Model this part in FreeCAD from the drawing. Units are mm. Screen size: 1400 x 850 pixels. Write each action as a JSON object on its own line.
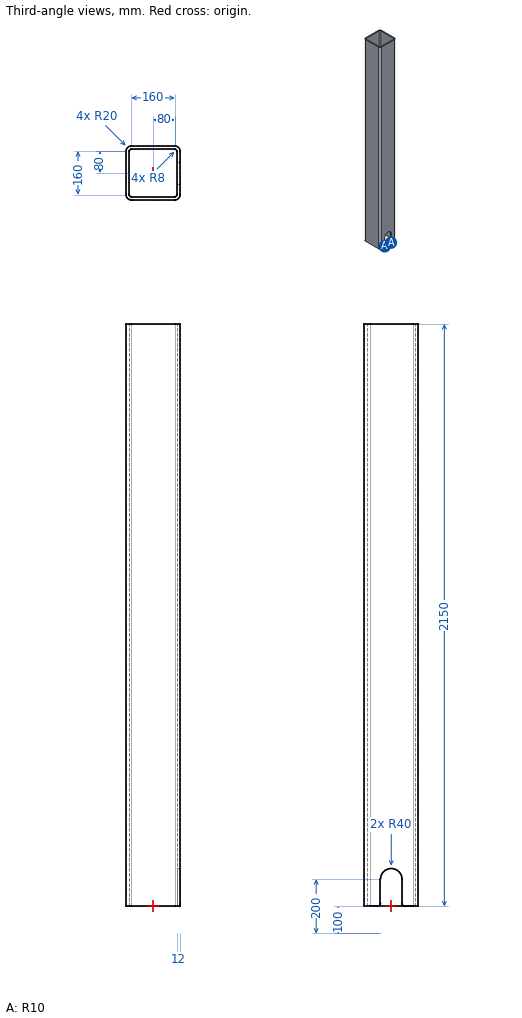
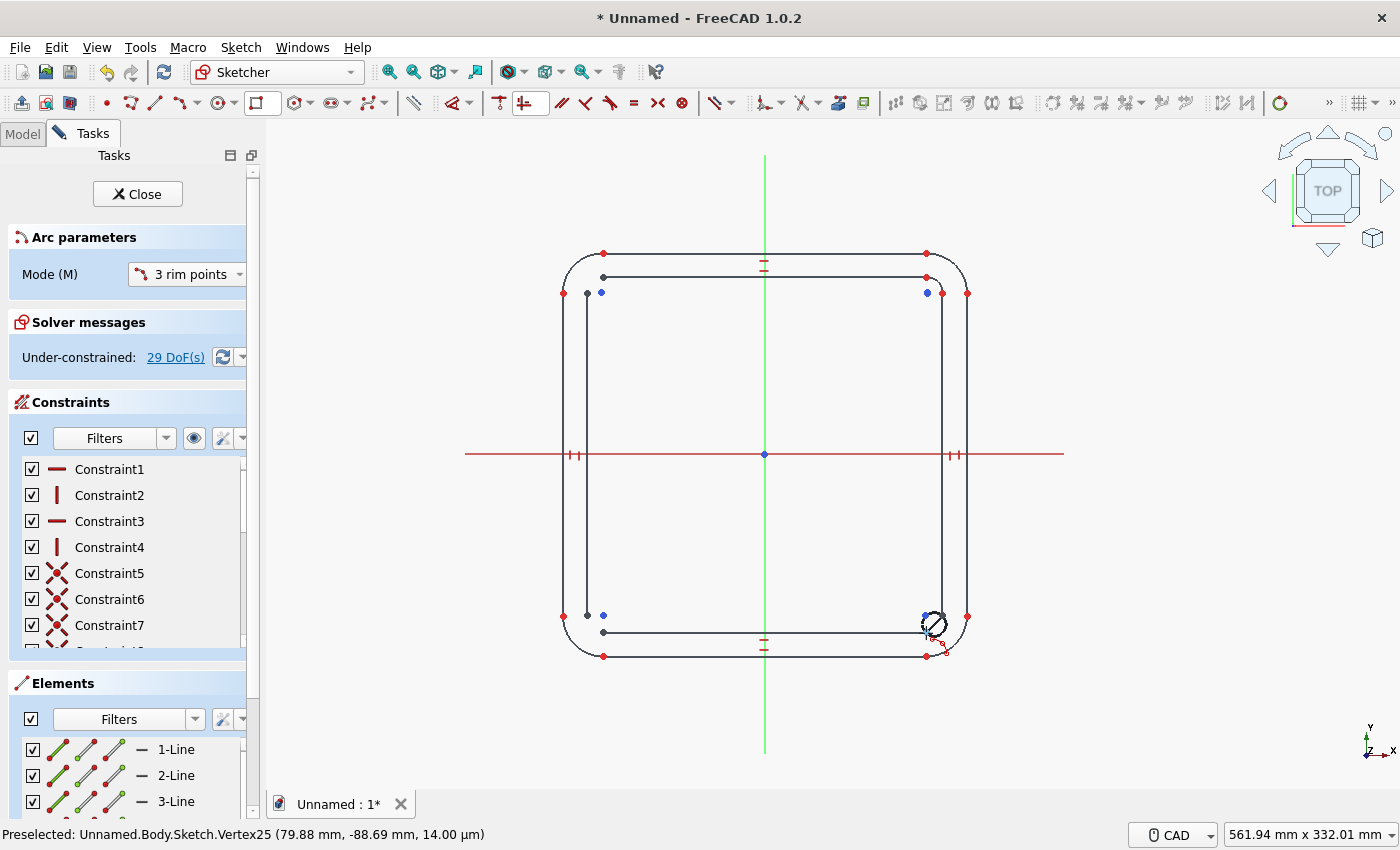
{"action": "scroll", "coordinate": [938, 627], "scroll_direction": "up", "scroll_amount": 7}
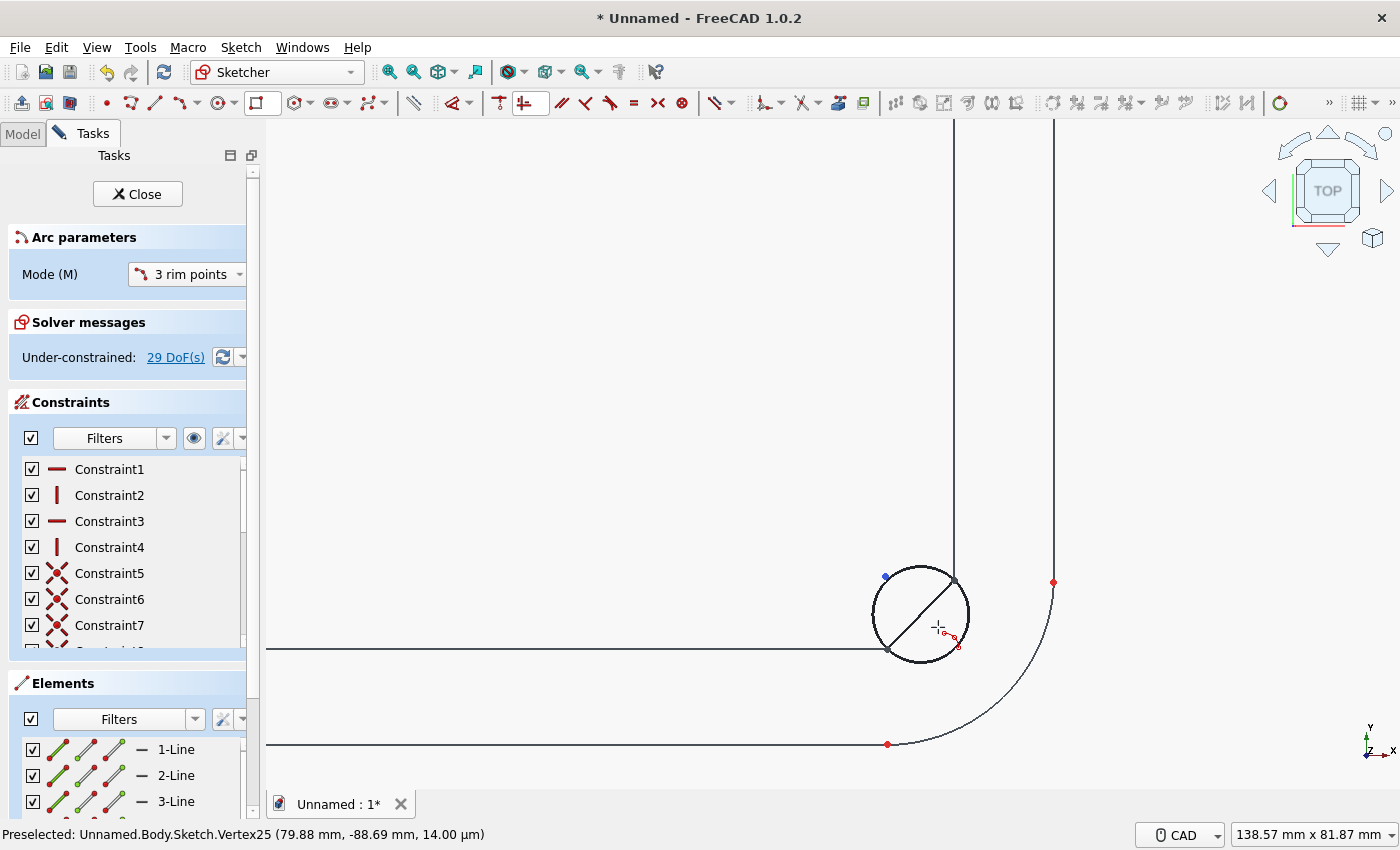
{"action": "left_click", "coordinate": [935, 624]}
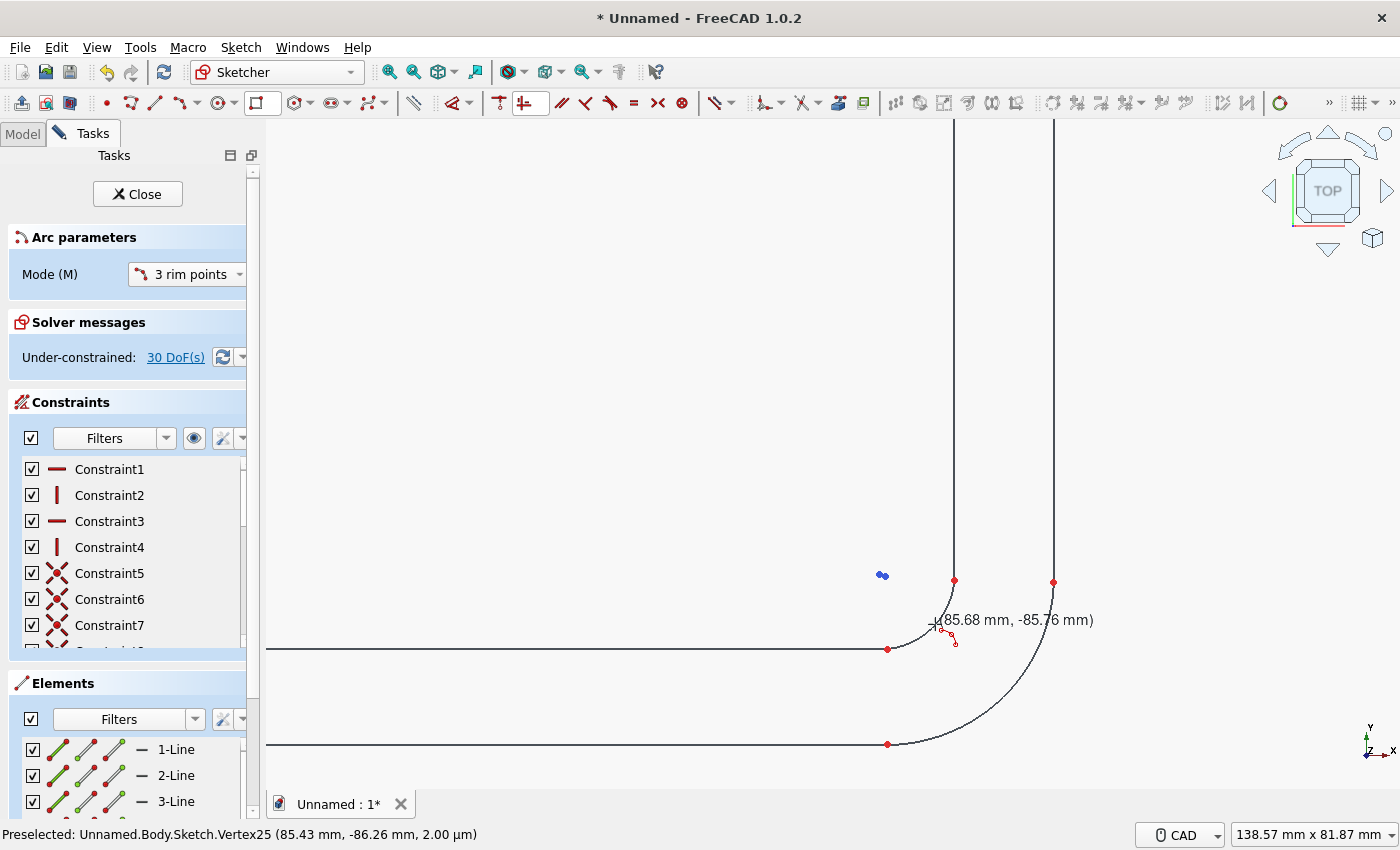
{"action": "scroll", "coordinate": [938, 628], "scroll_direction": "down", "scroll_amount": 7}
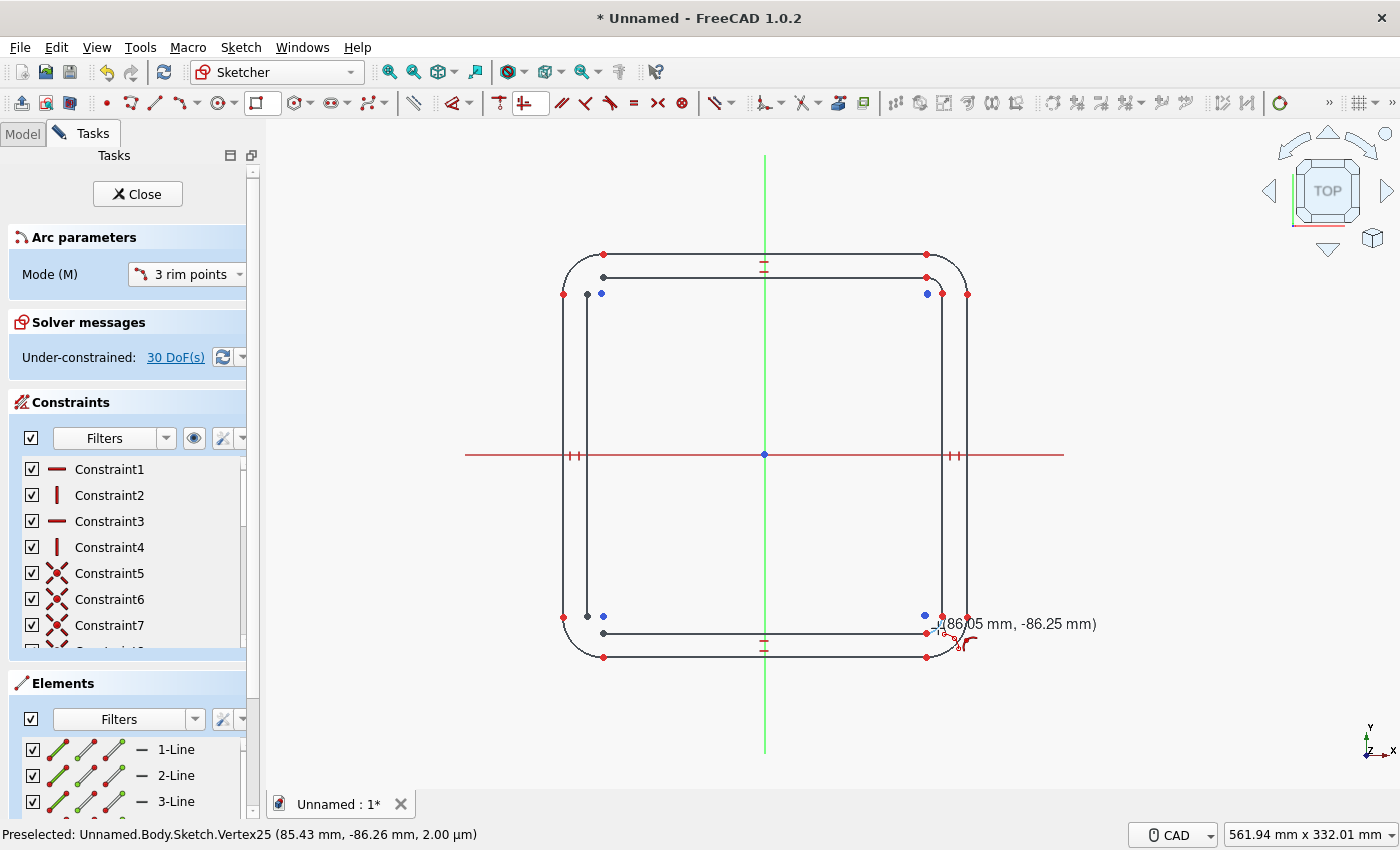
{"action": "left_click", "coordinate": [603, 634]}
{"action": "left_click", "coordinate": [587, 617]}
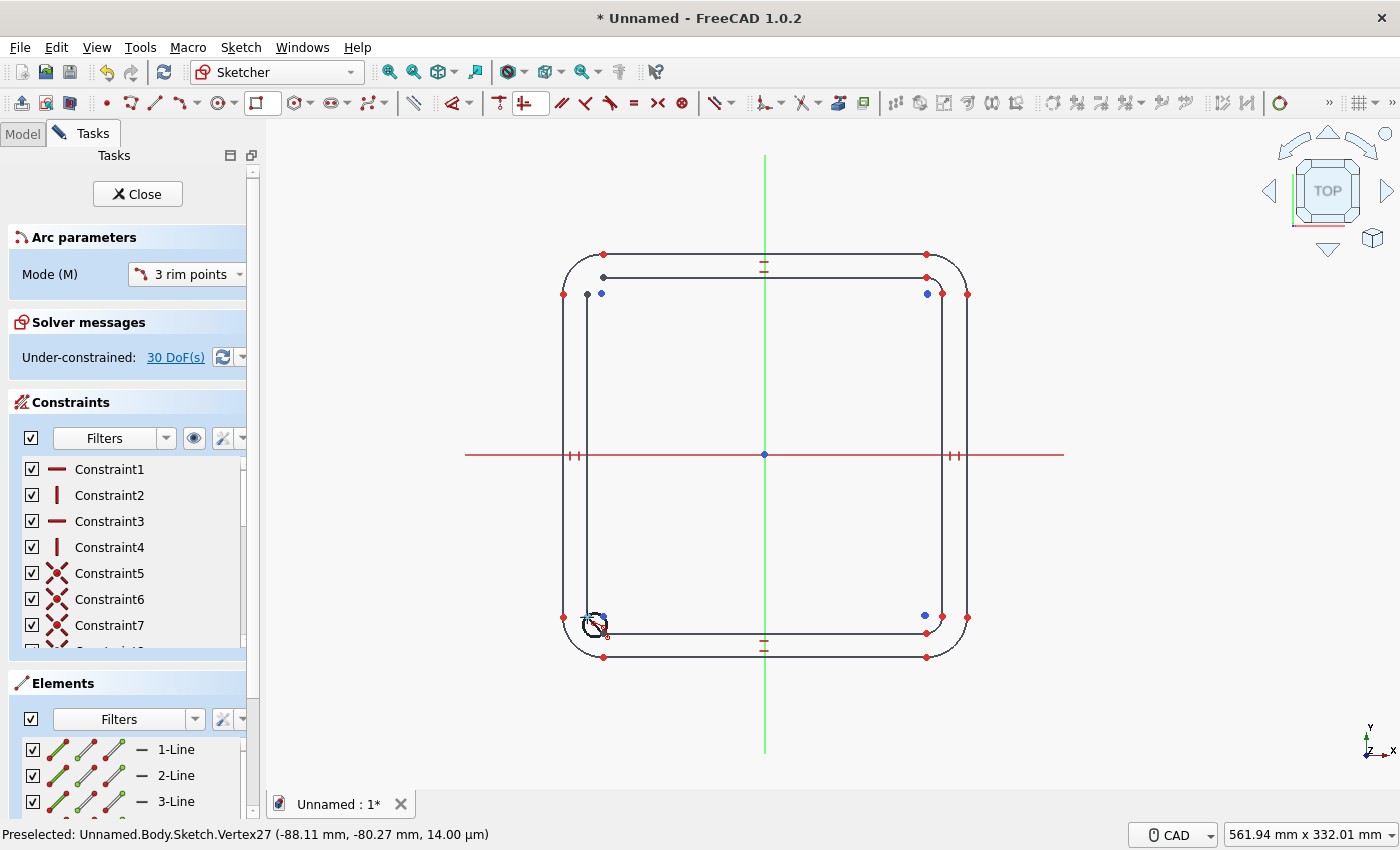
{"action": "scroll", "coordinate": [592, 628], "scroll_direction": "up", "scroll_amount": 7}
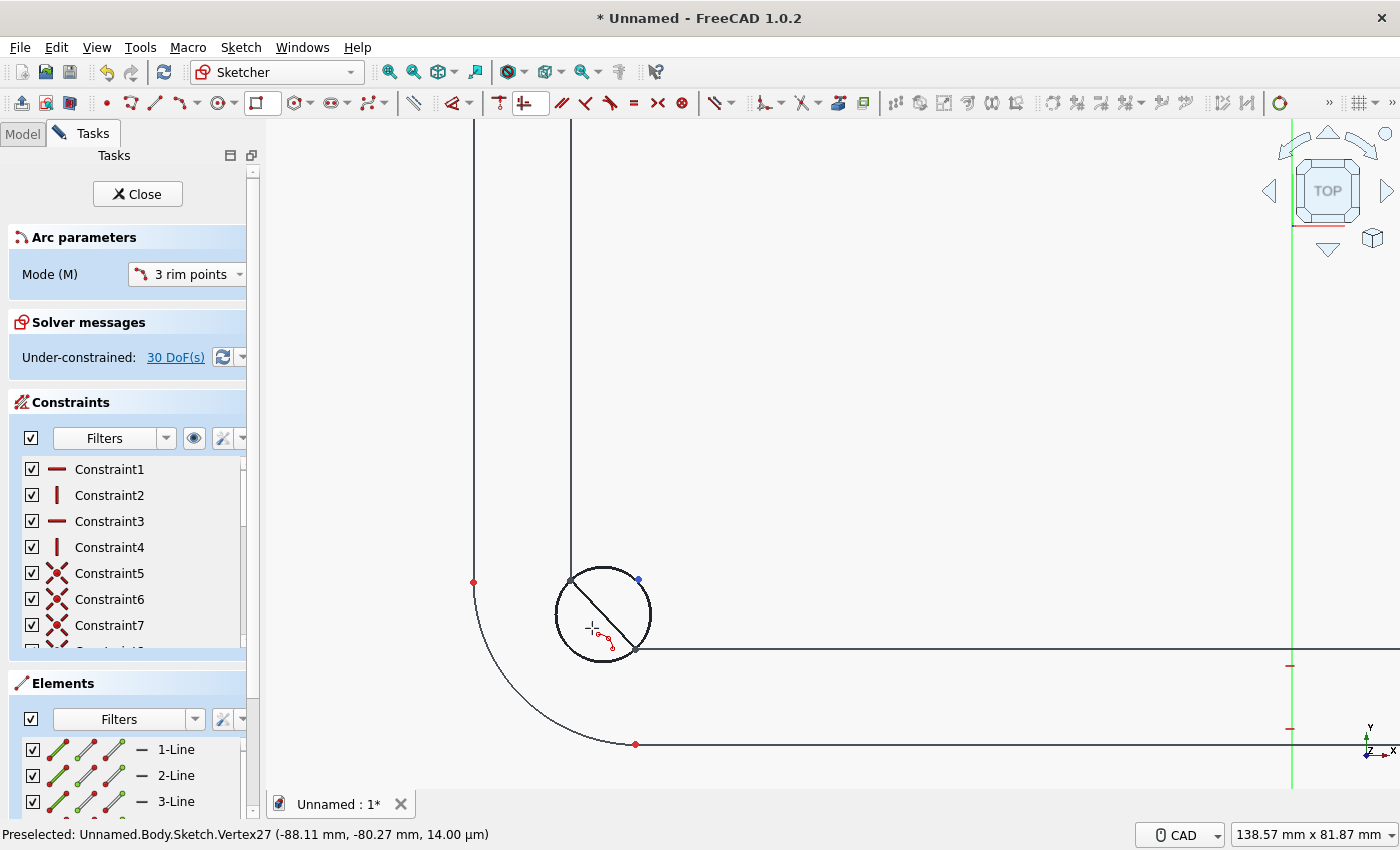
{"action": "left_click", "coordinate": [591, 624]}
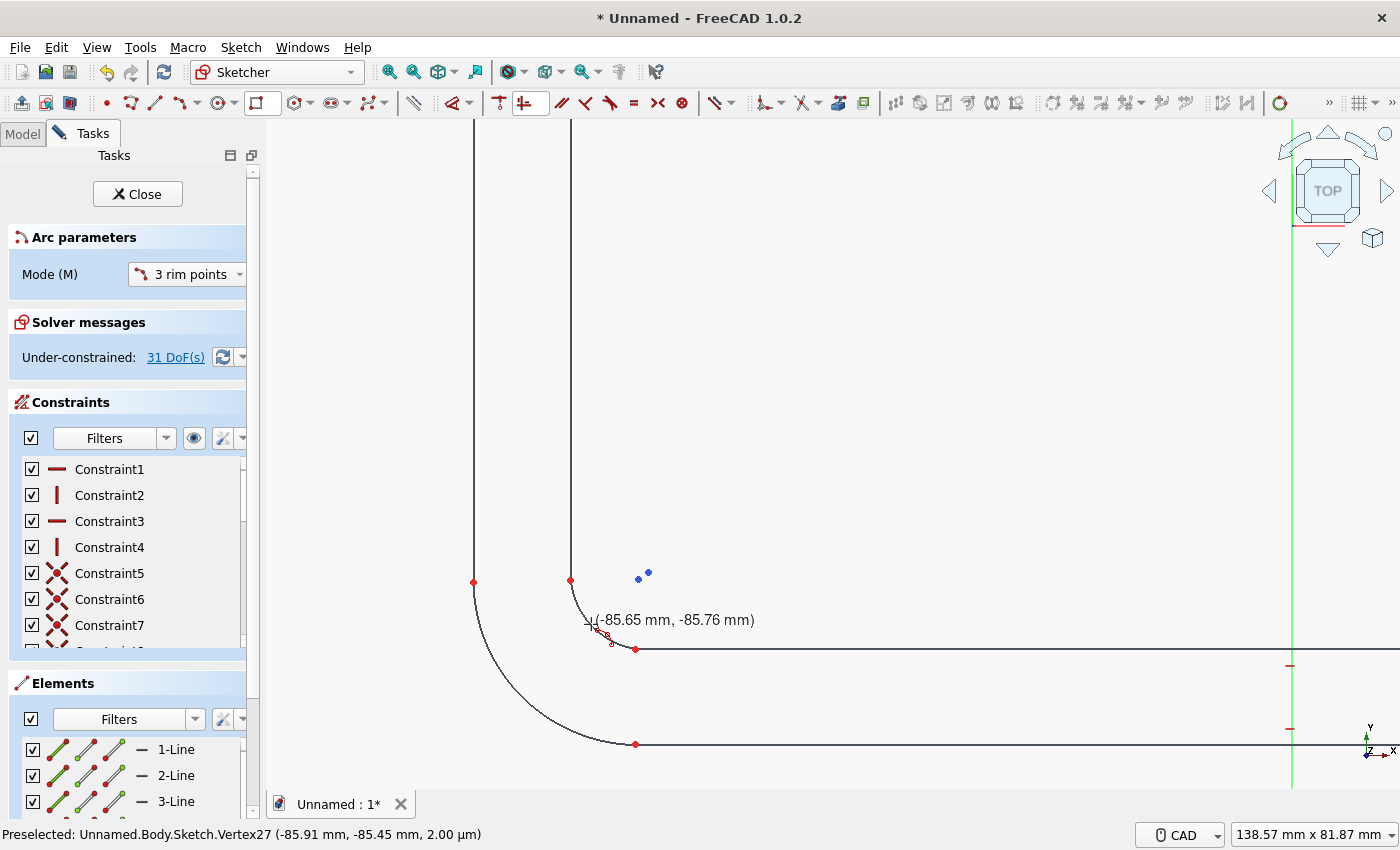
{"action": "scroll", "coordinate": [592, 628], "scroll_direction": "down", "scroll_amount": 7}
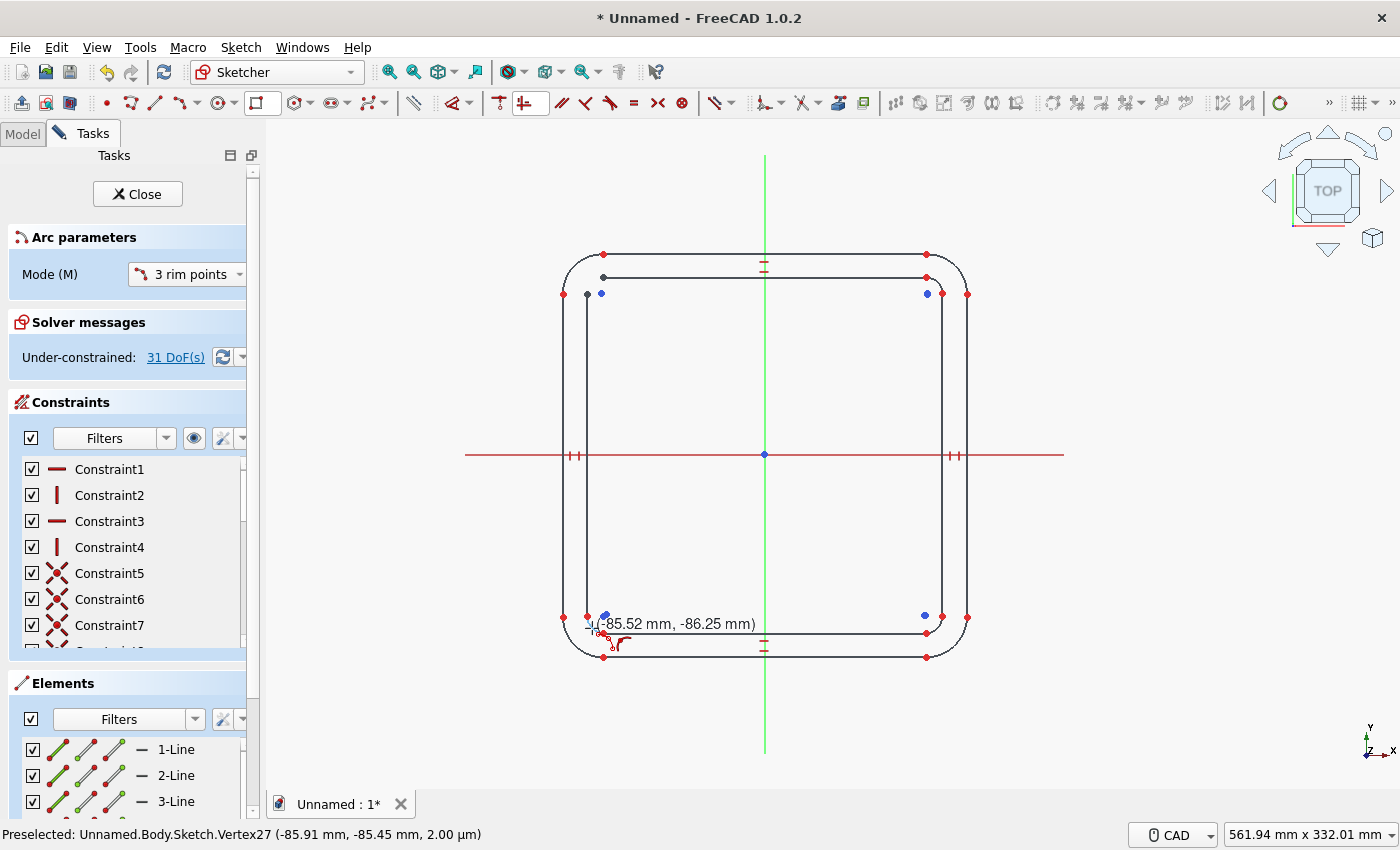
{"action": "left_click", "coordinate": [587, 295]}
{"action": "left_click", "coordinate": [603, 278]}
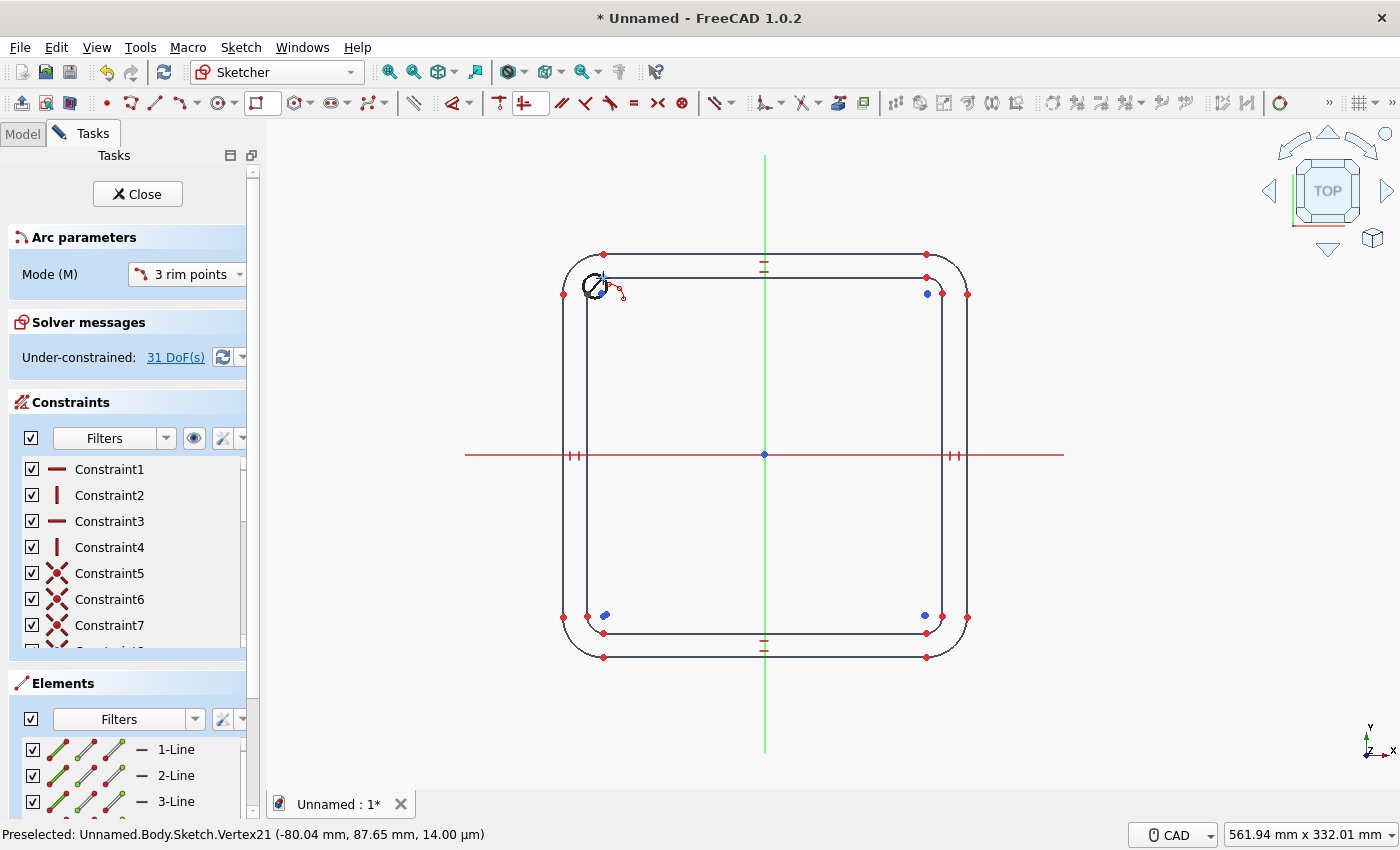
{"action": "scroll", "coordinate": [592, 282], "scroll_direction": "up", "scroll_amount": 7}